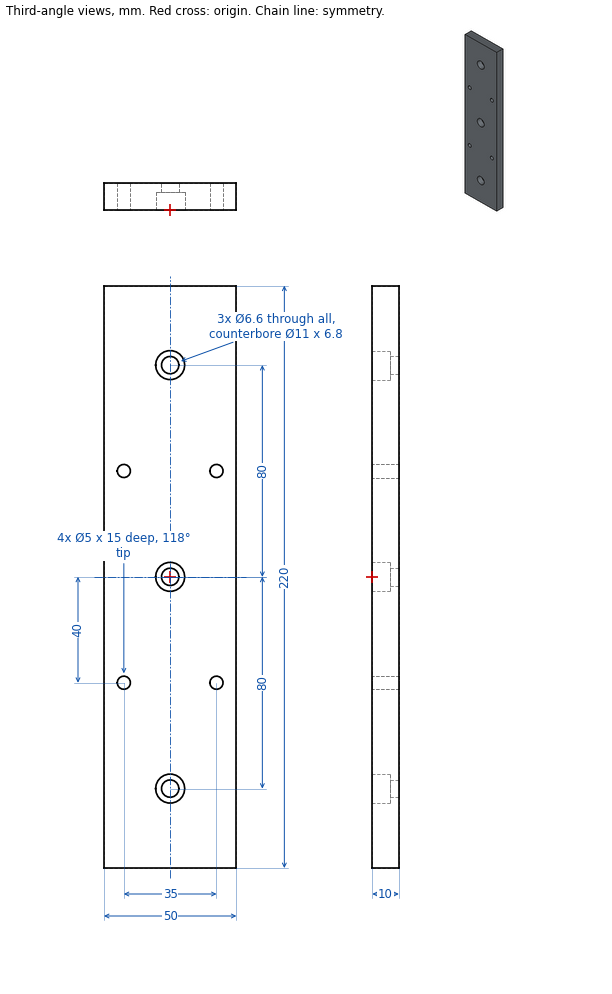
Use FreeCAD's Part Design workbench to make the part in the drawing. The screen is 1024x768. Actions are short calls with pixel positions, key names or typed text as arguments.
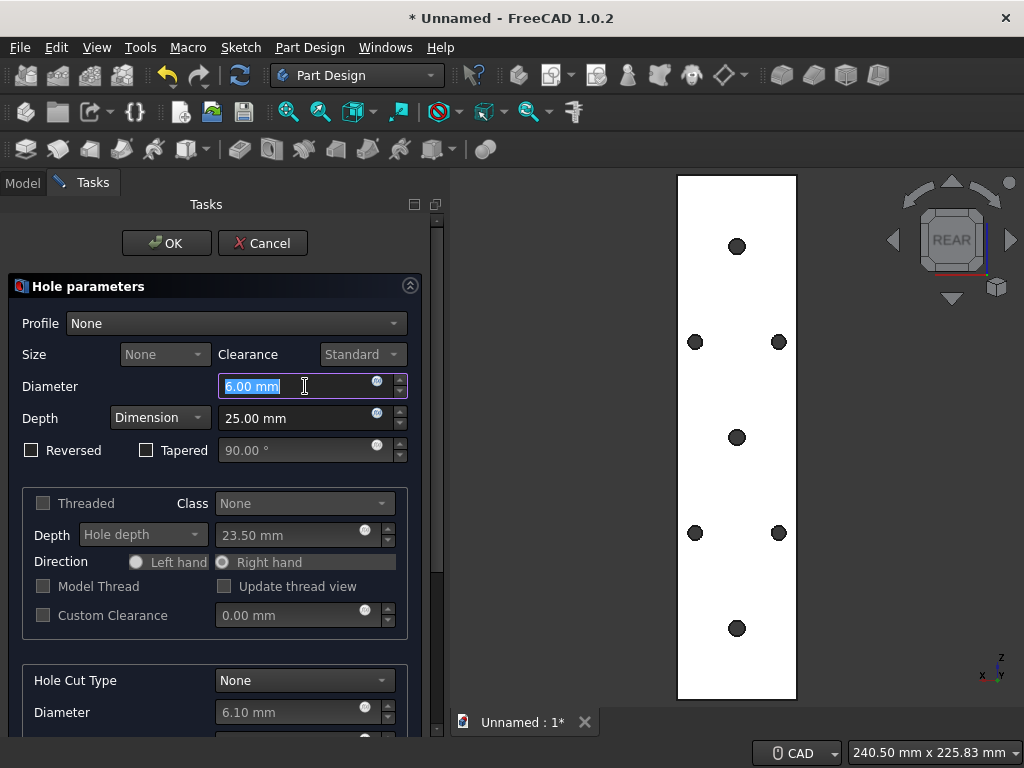
text(5)
key(Tab)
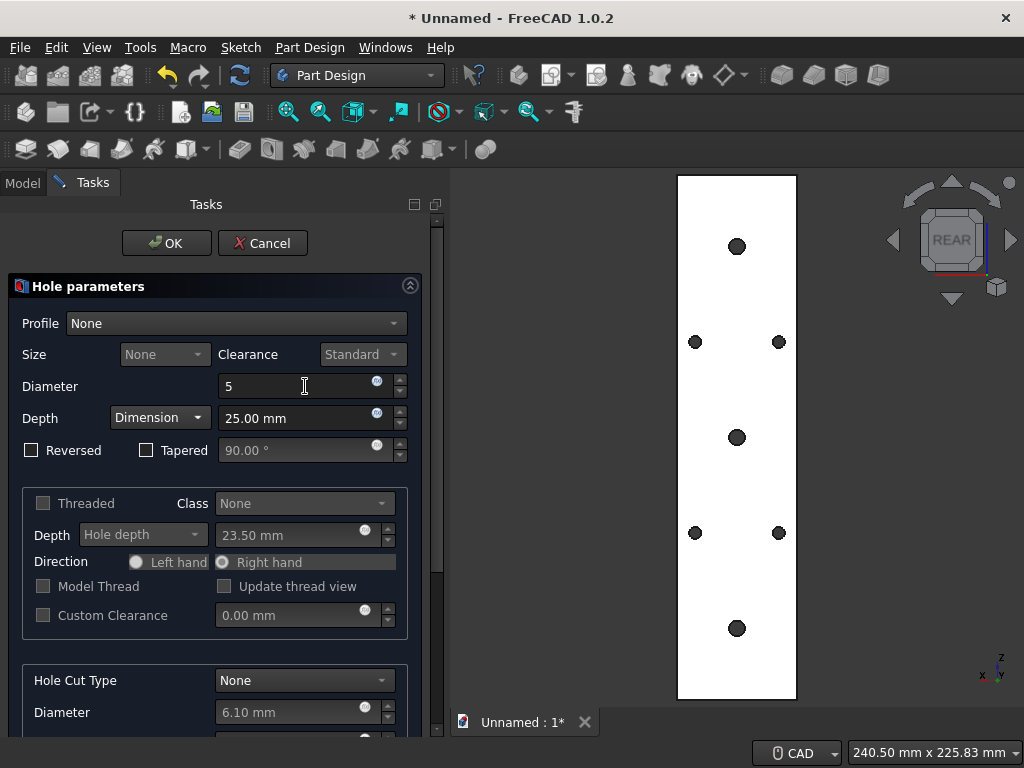
triple_click(305, 418)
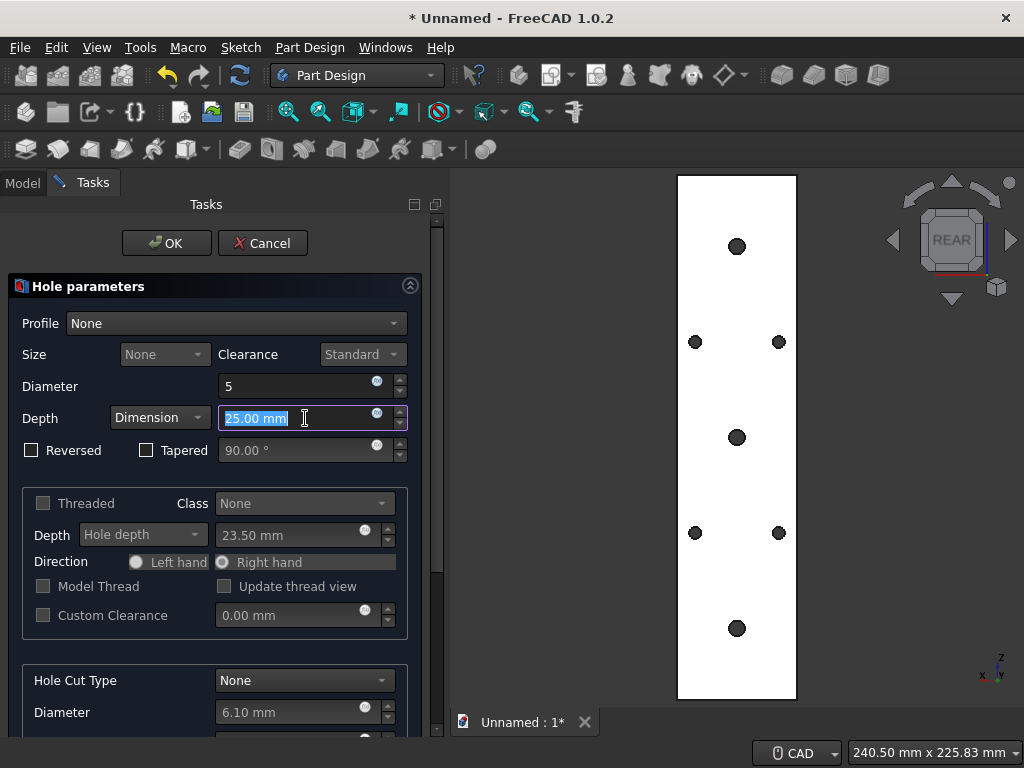
text(15)
key(Tab)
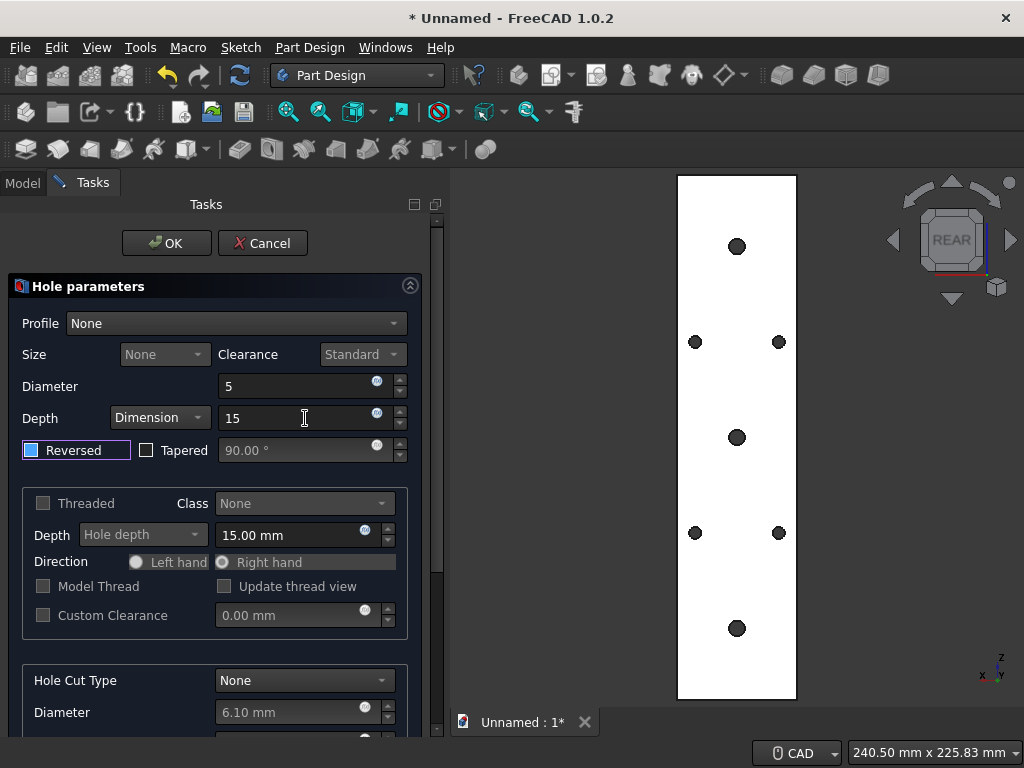
click(167, 243)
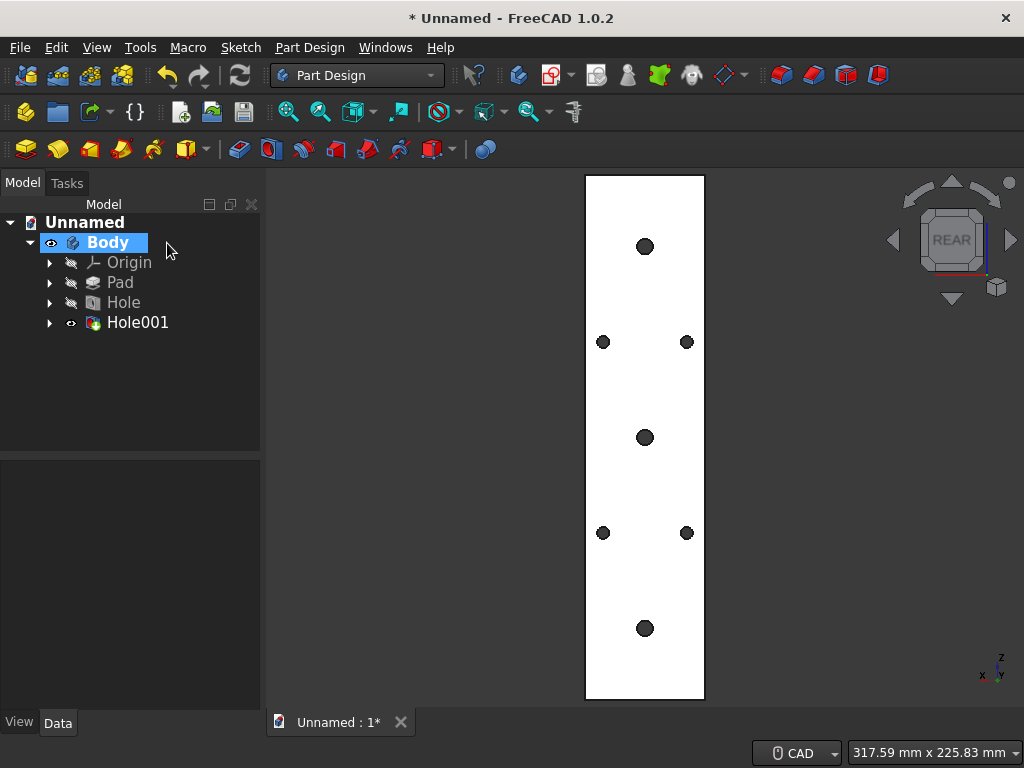
key(0)